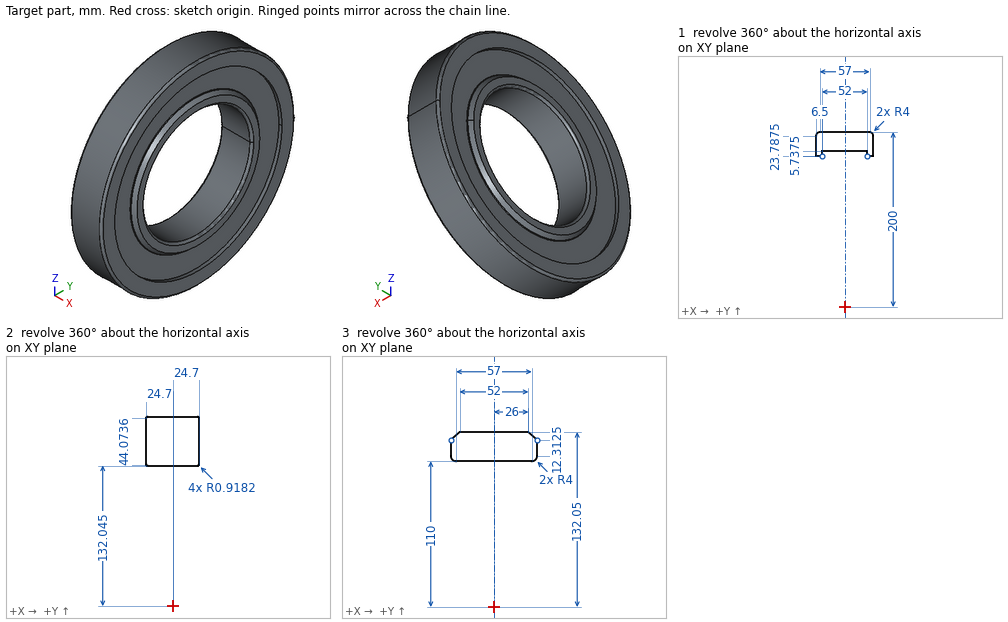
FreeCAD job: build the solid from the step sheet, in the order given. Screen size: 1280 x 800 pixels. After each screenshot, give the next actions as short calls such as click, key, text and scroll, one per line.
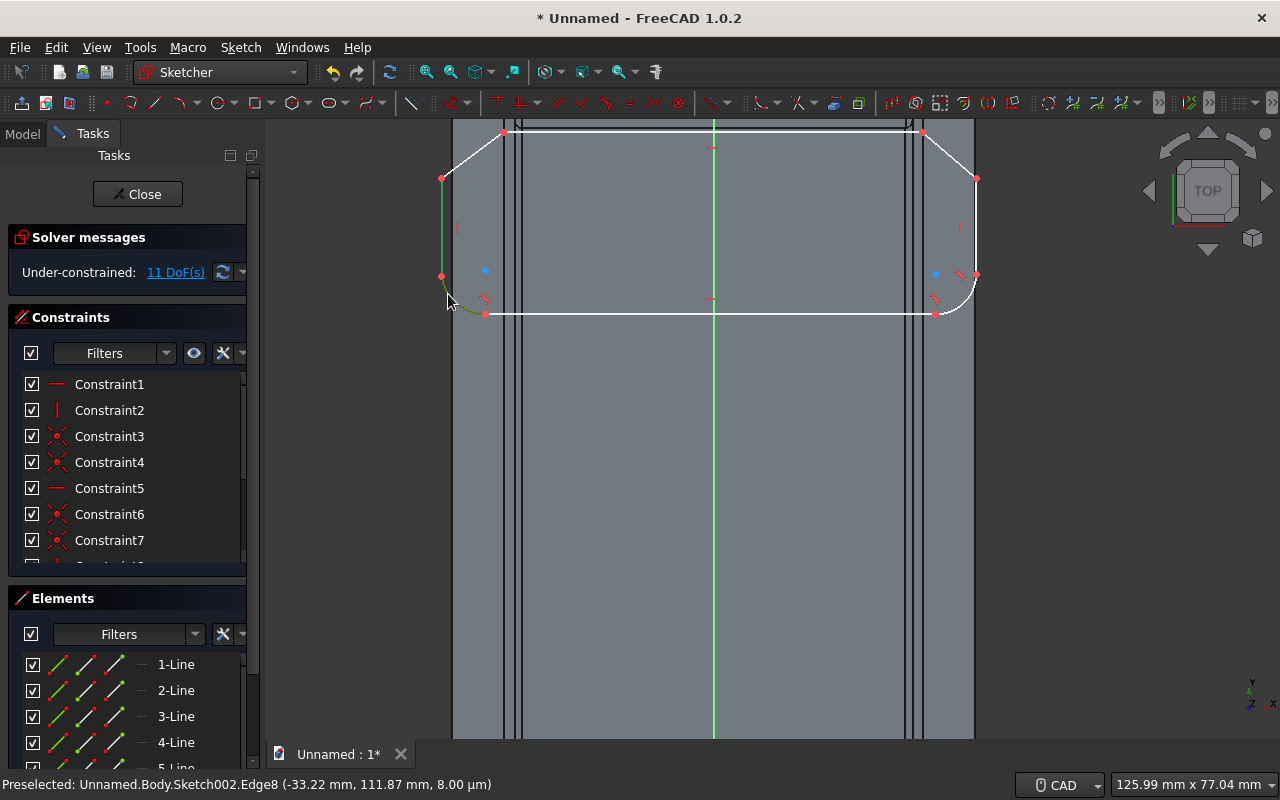
click(606, 104)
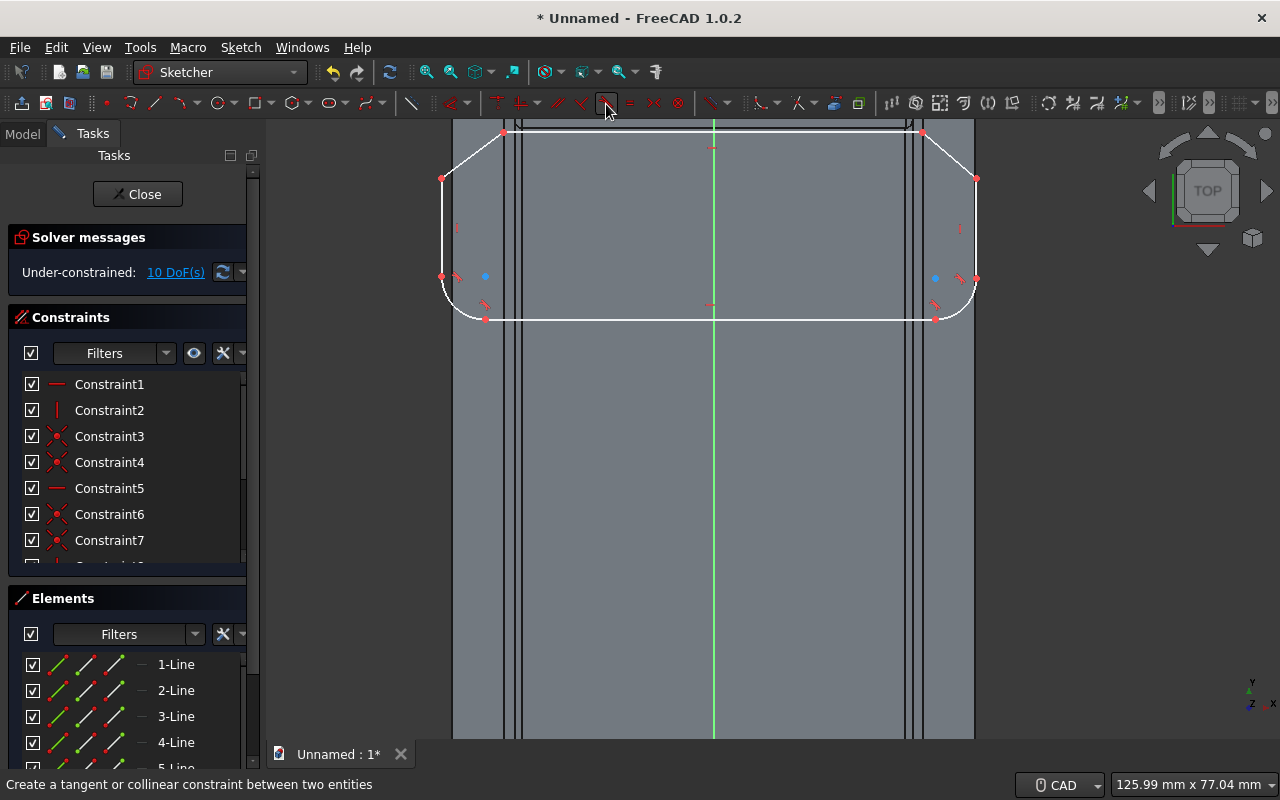
click(954, 315)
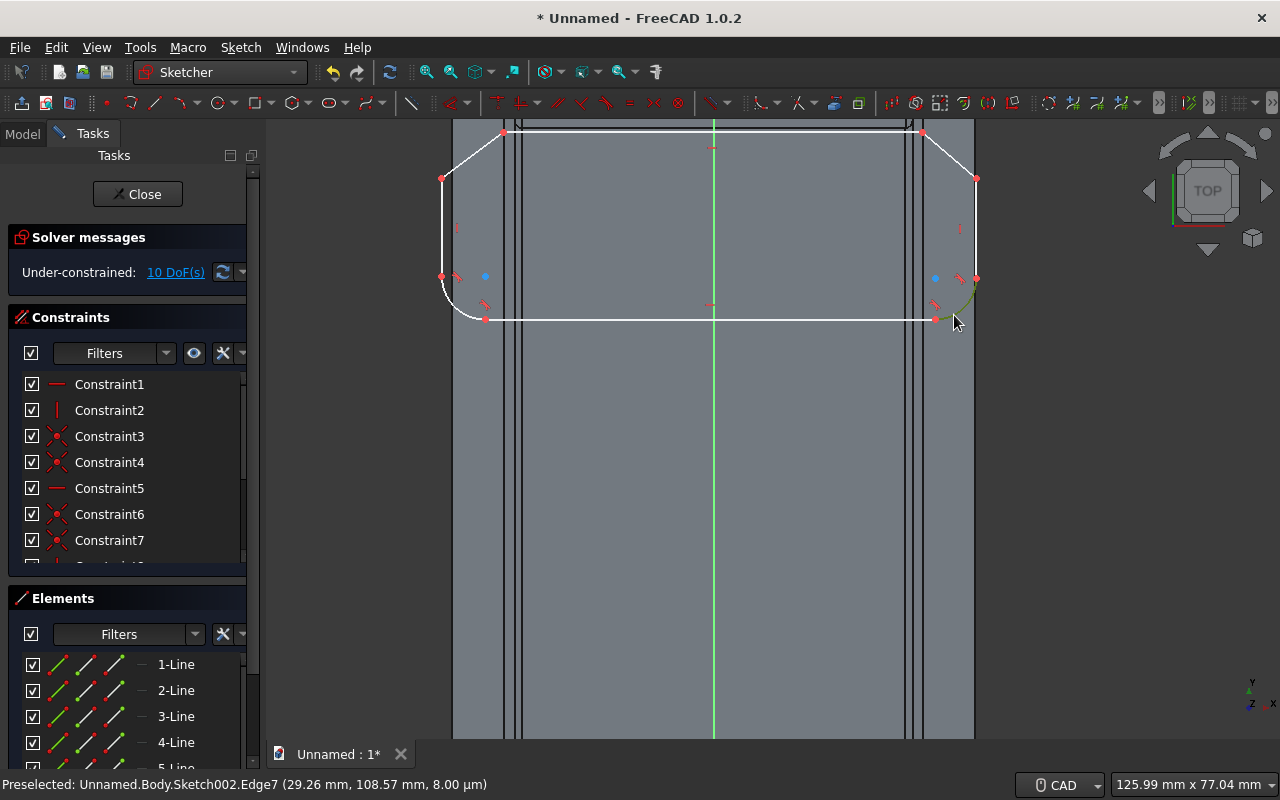
click(447, 296)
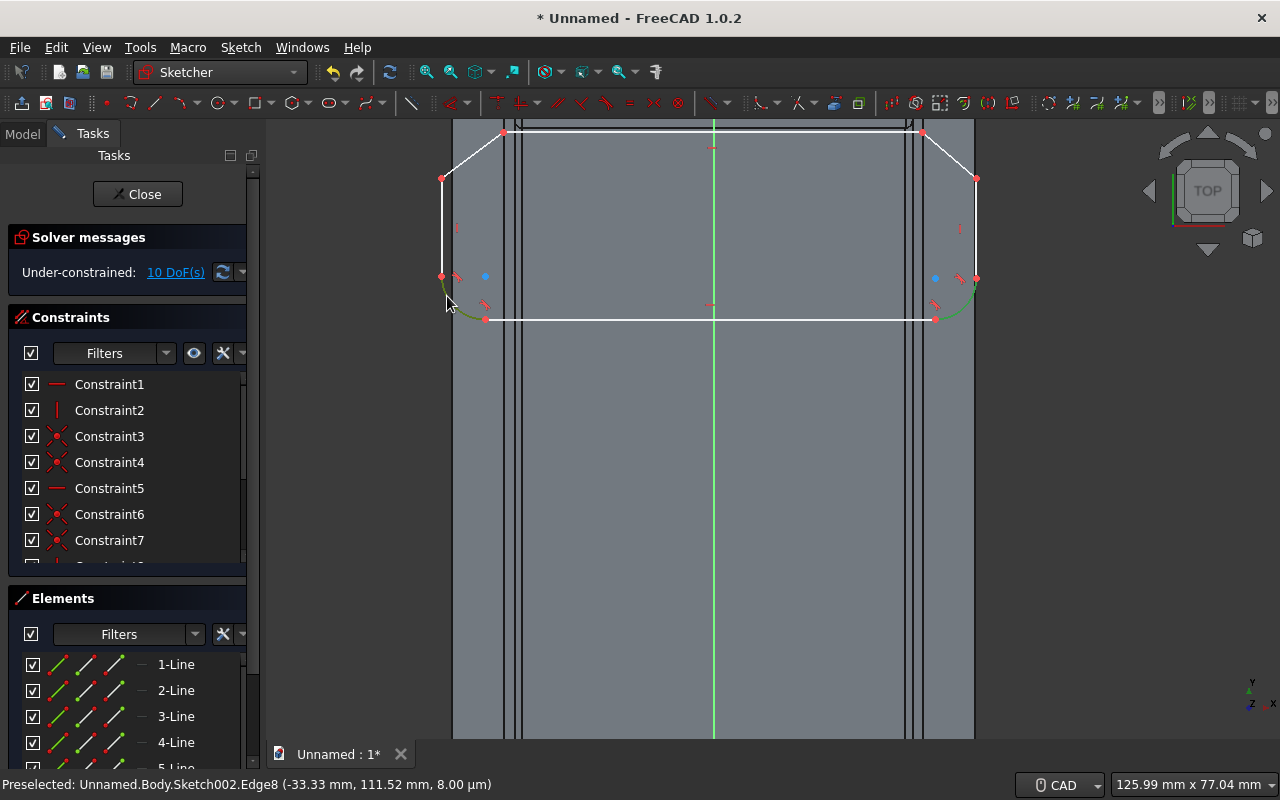
click(630, 104)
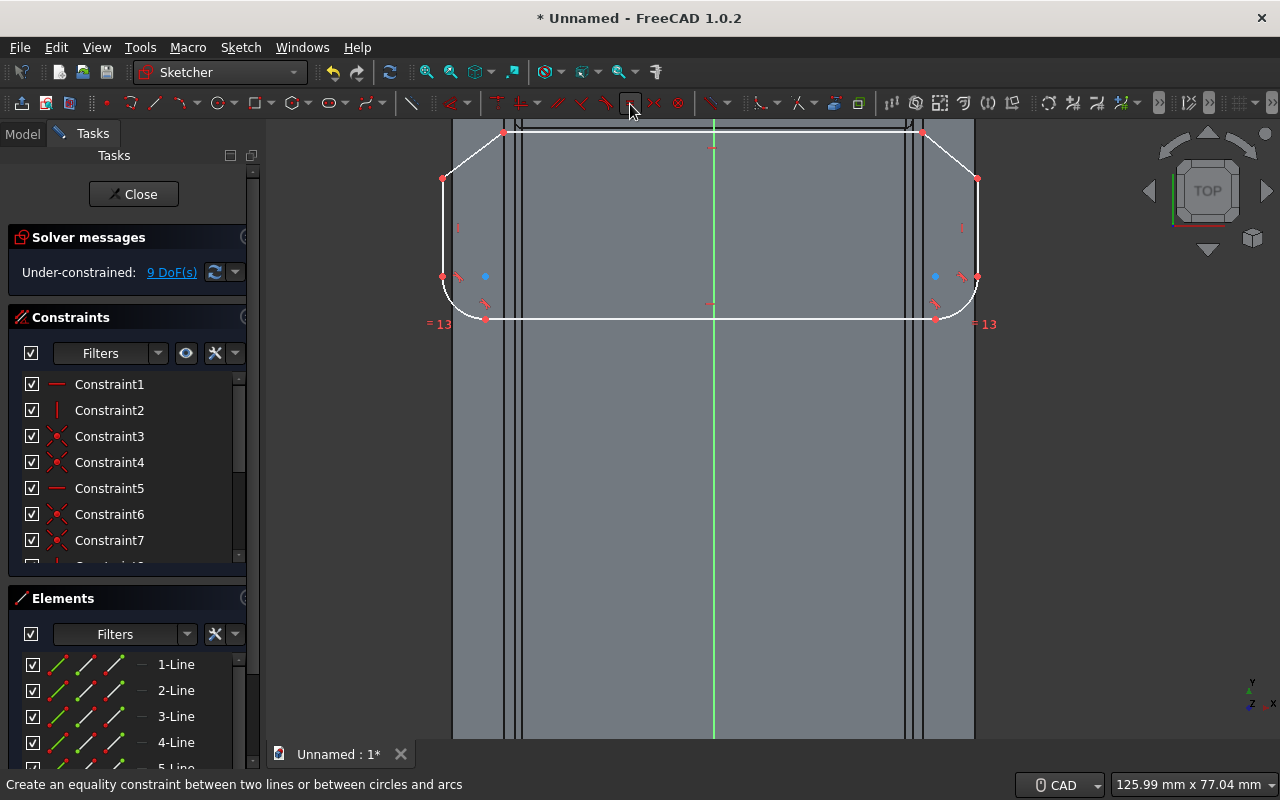
click(978, 178)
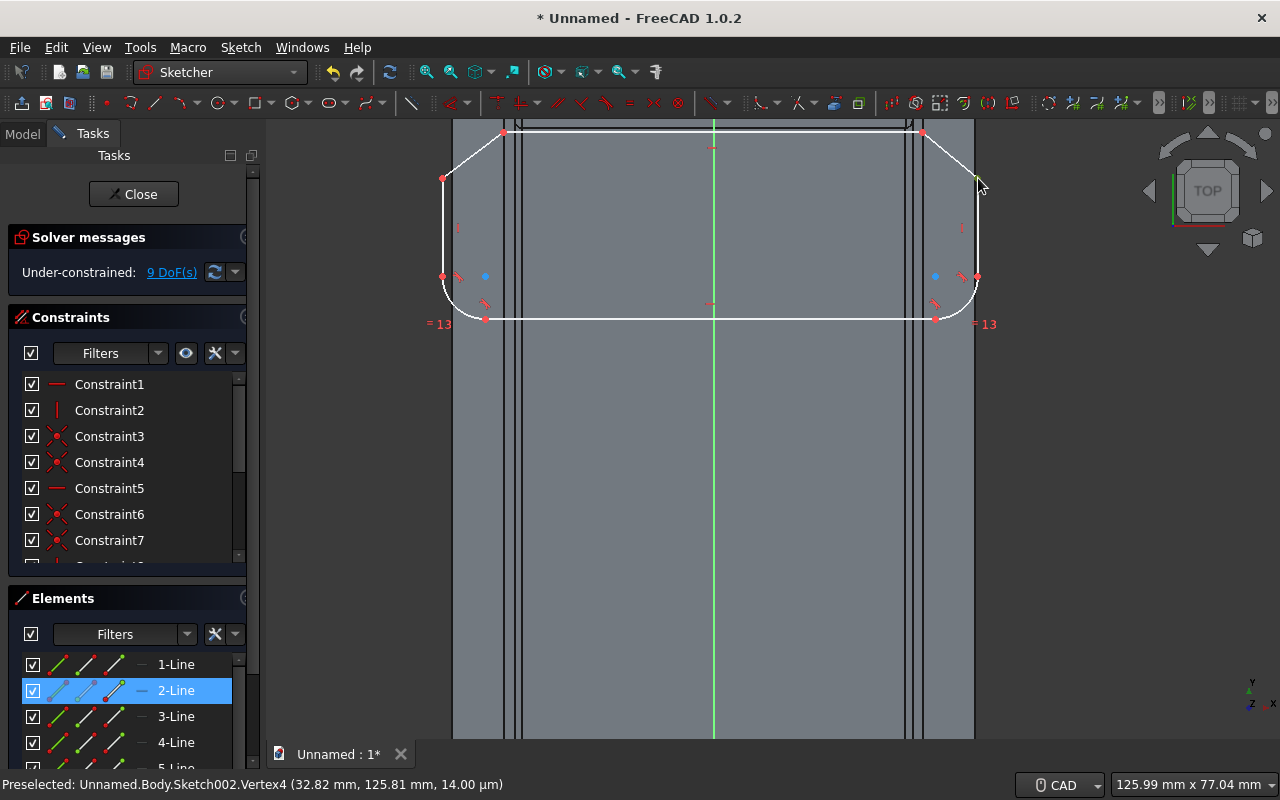
click(443, 178)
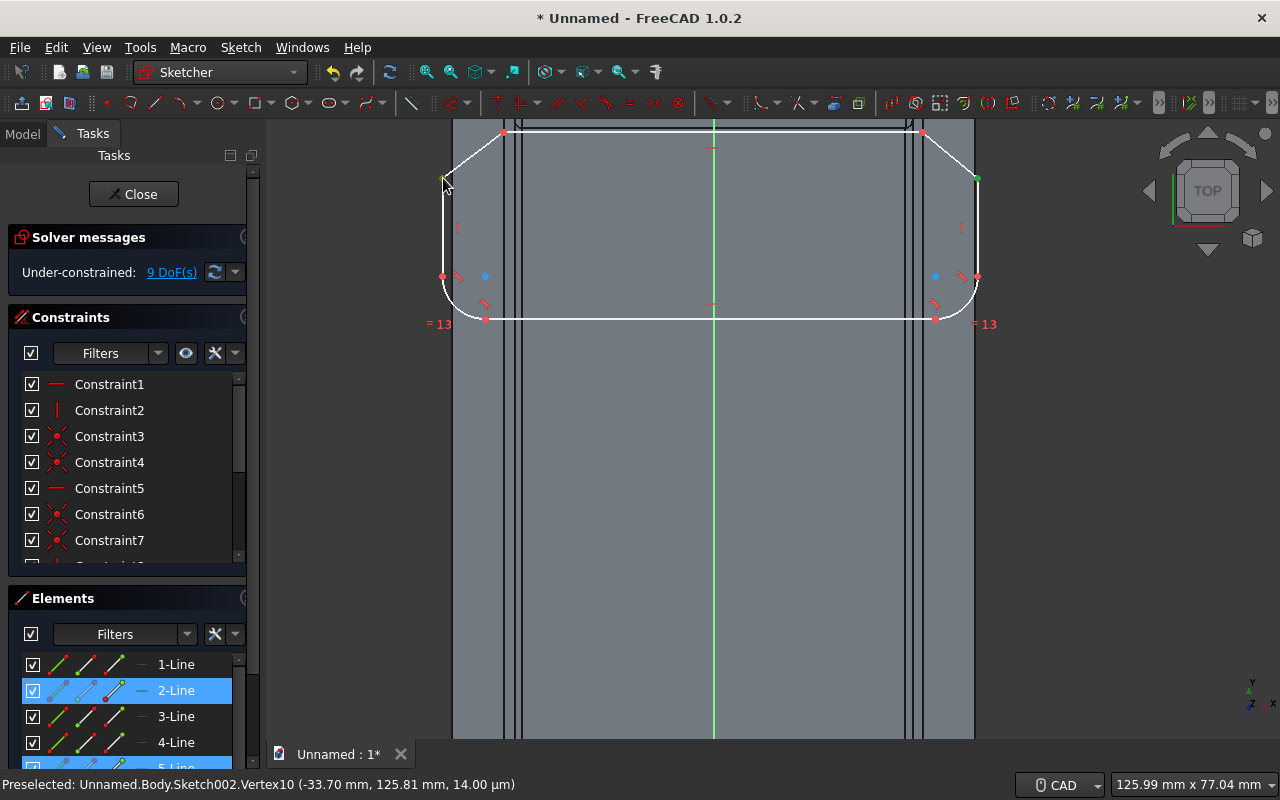
click(714, 671)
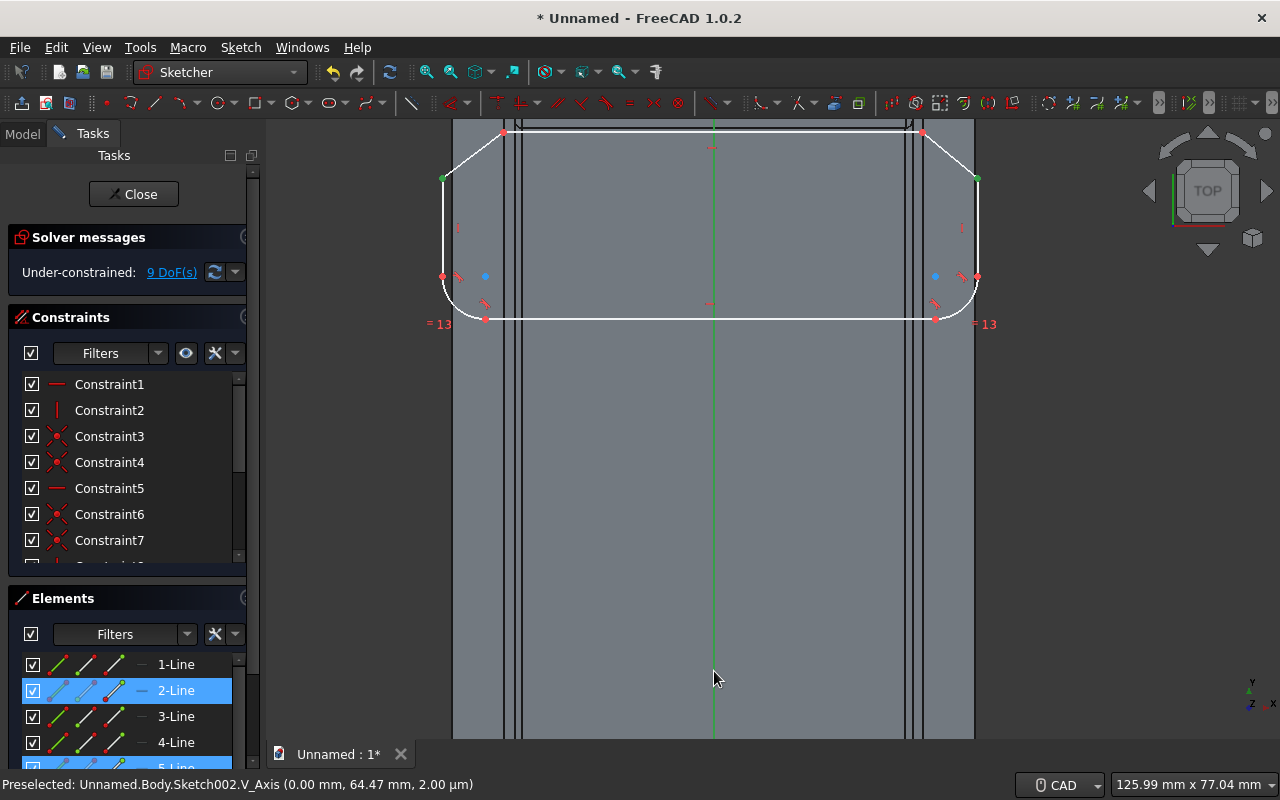
click(654, 104)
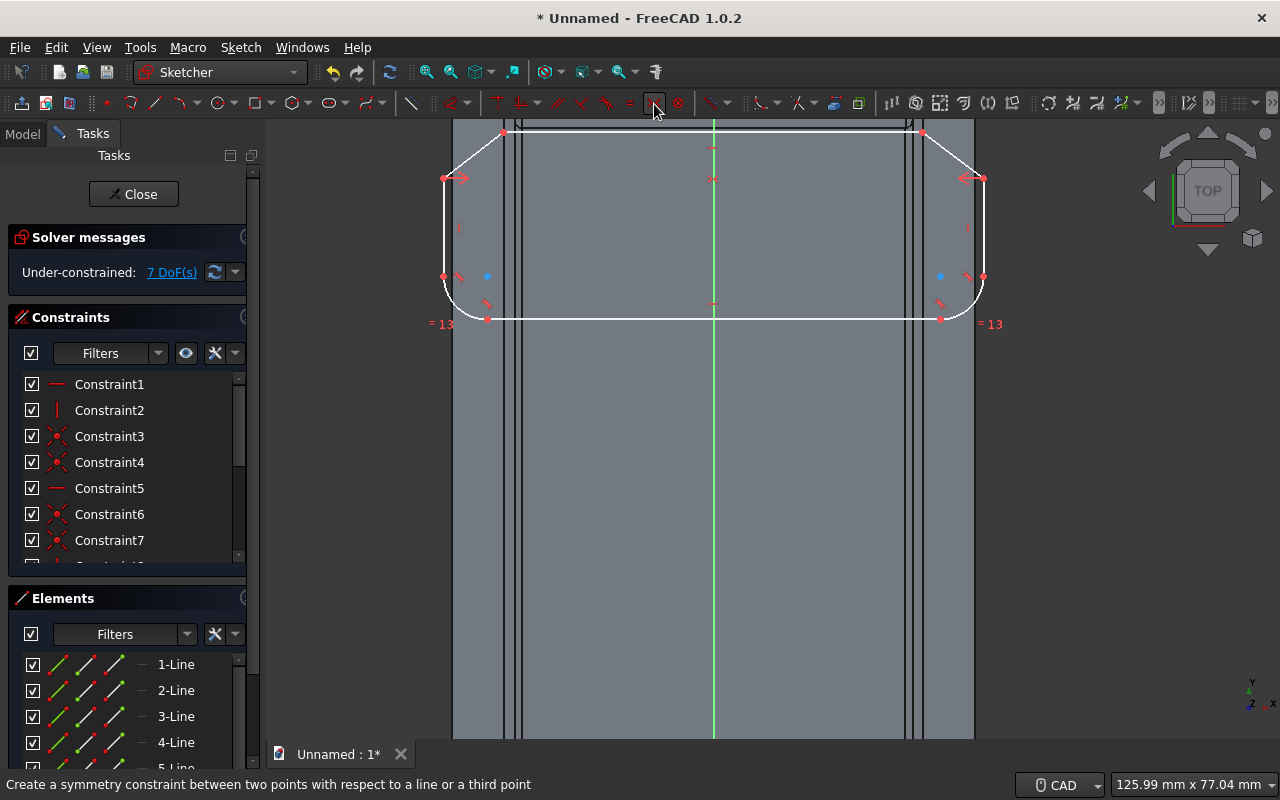
click(450, 104)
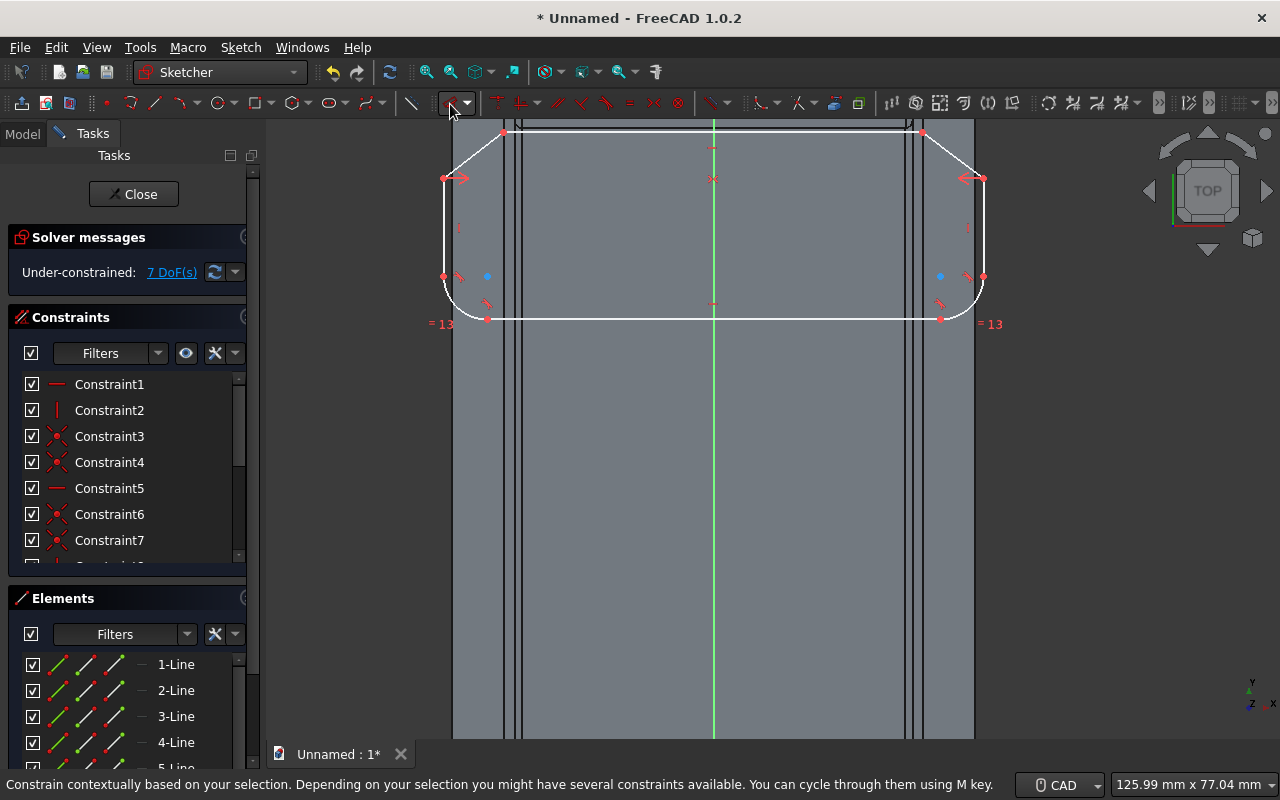
scroll(960, 315, up, 2)